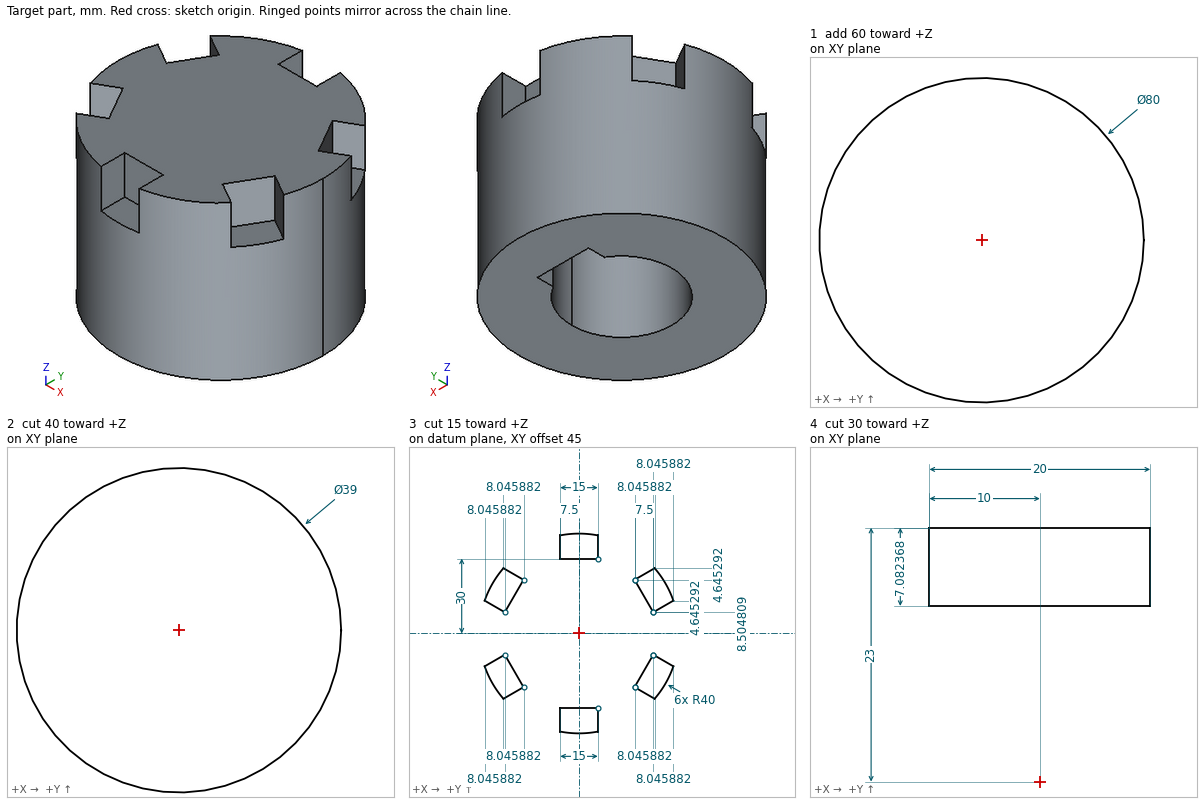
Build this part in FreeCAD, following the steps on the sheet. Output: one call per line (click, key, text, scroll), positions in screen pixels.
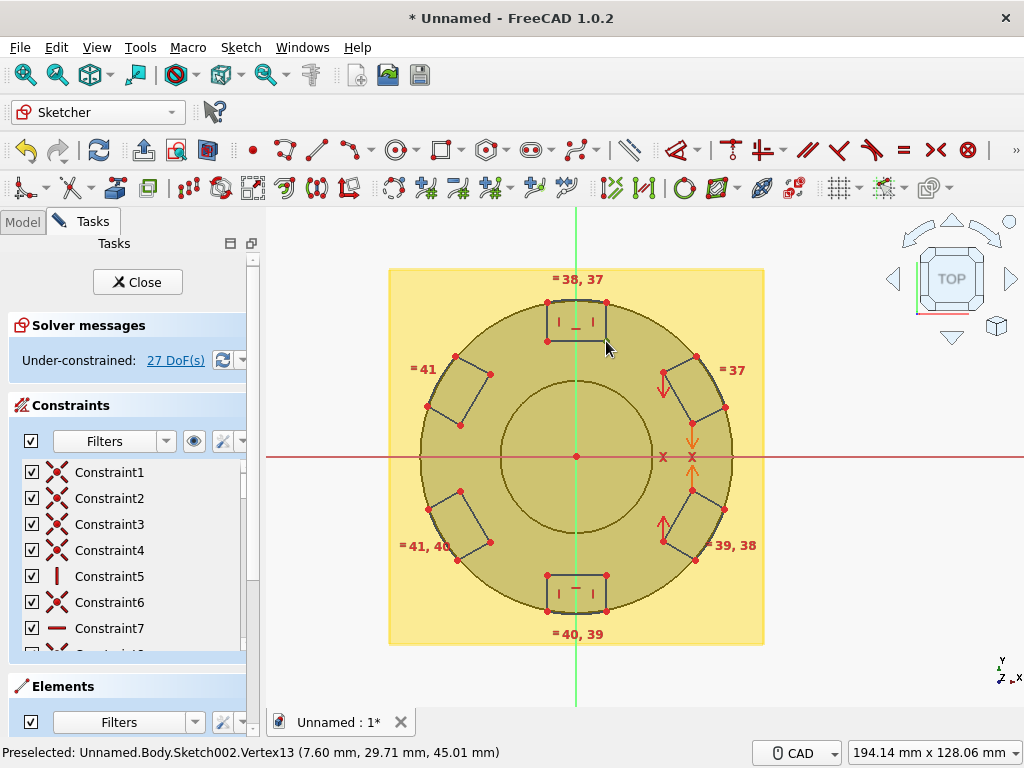
click(606, 575)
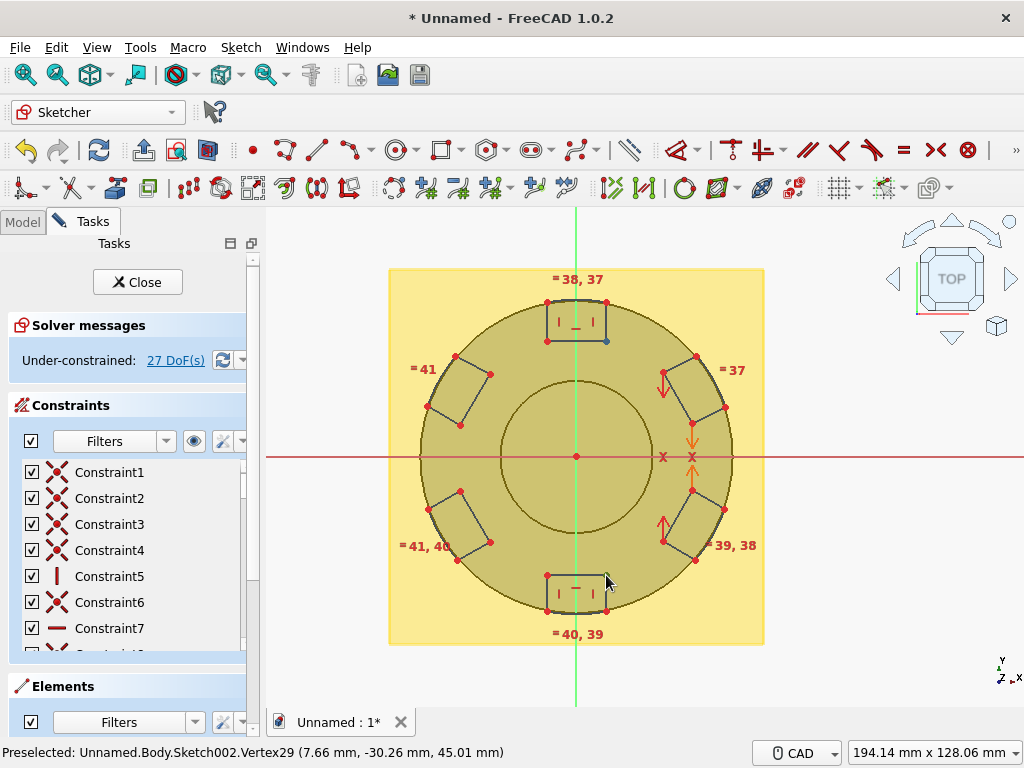
click(334, 457)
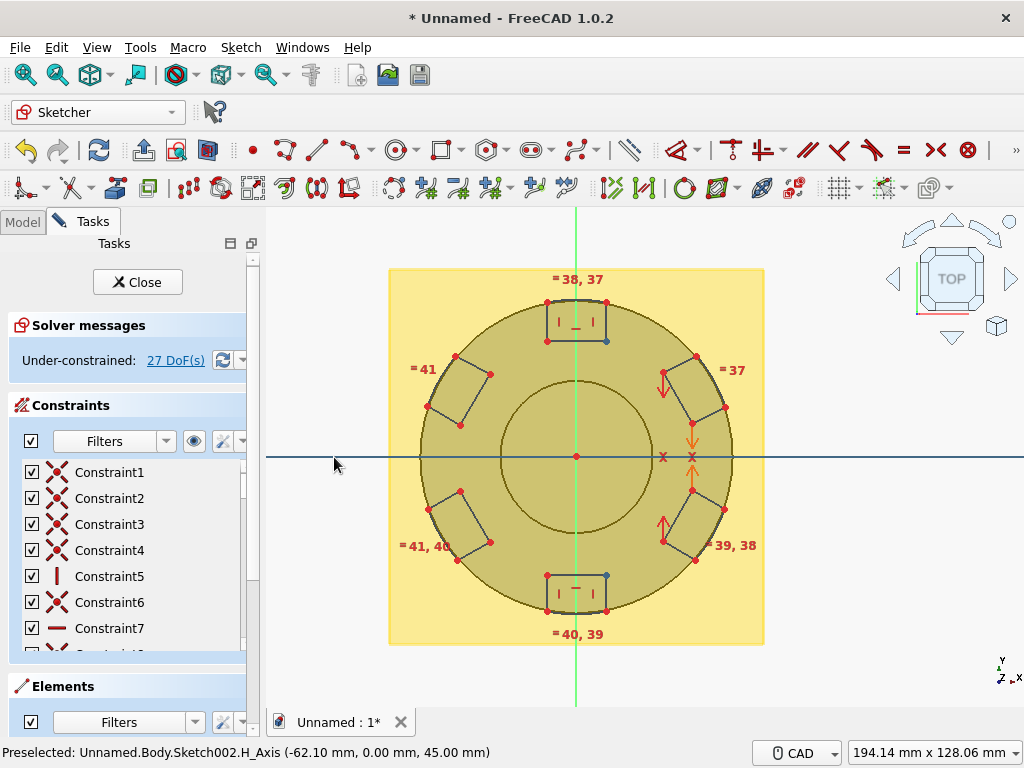
click(936, 150)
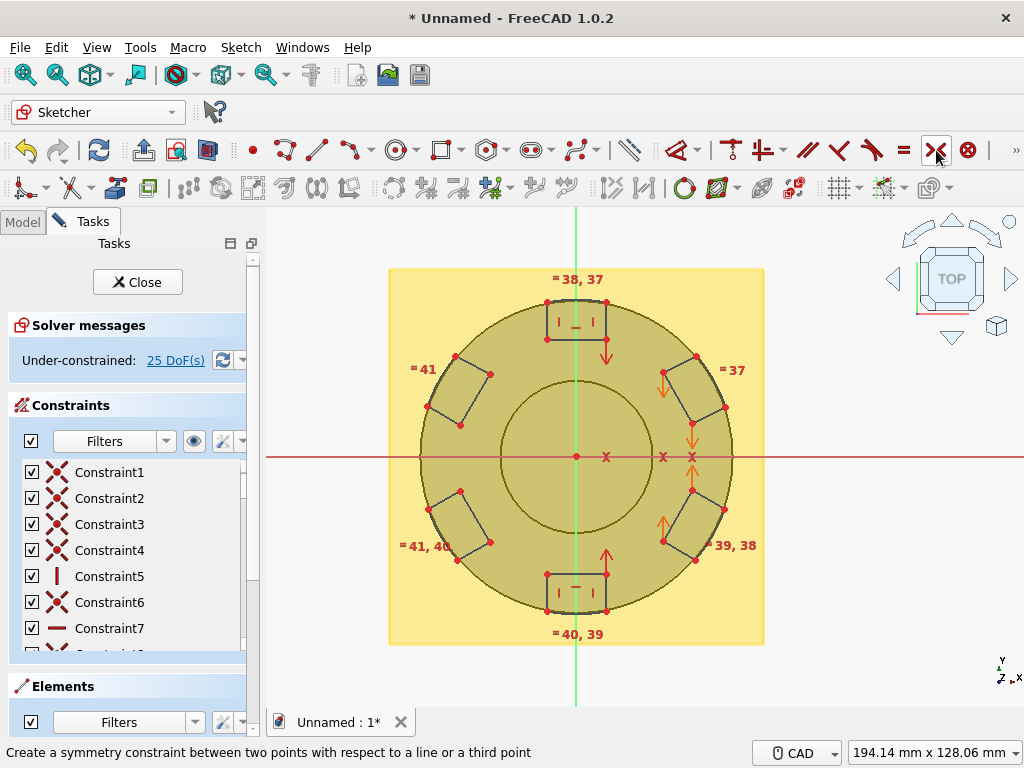
click(663, 541)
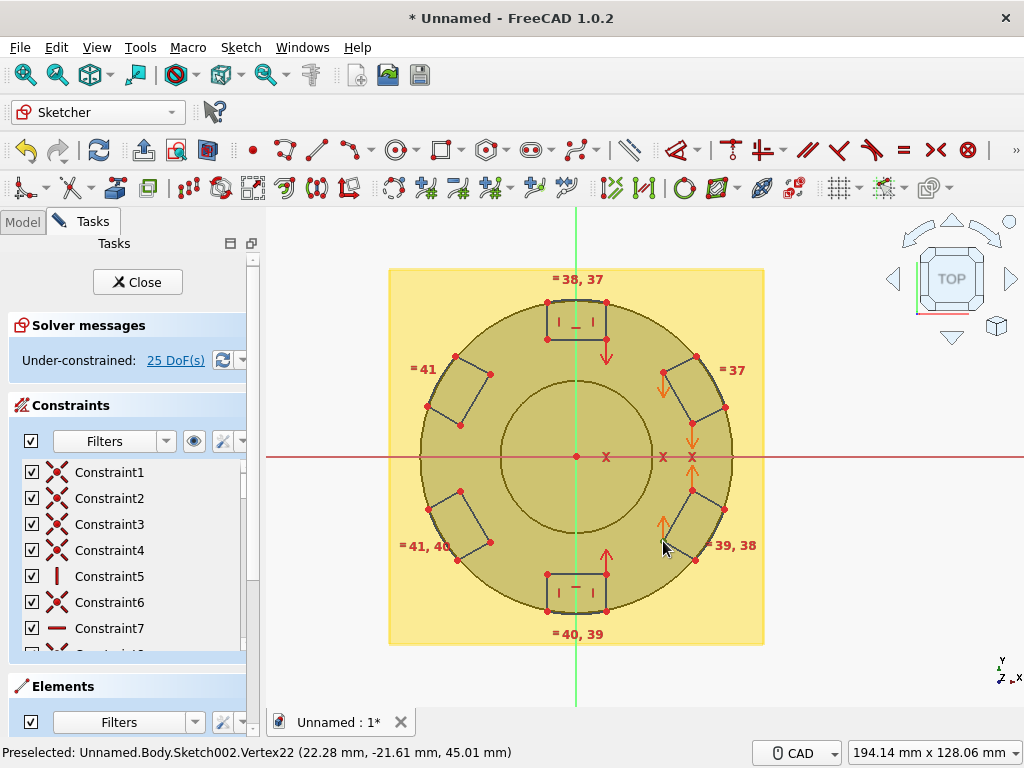
click(490, 542)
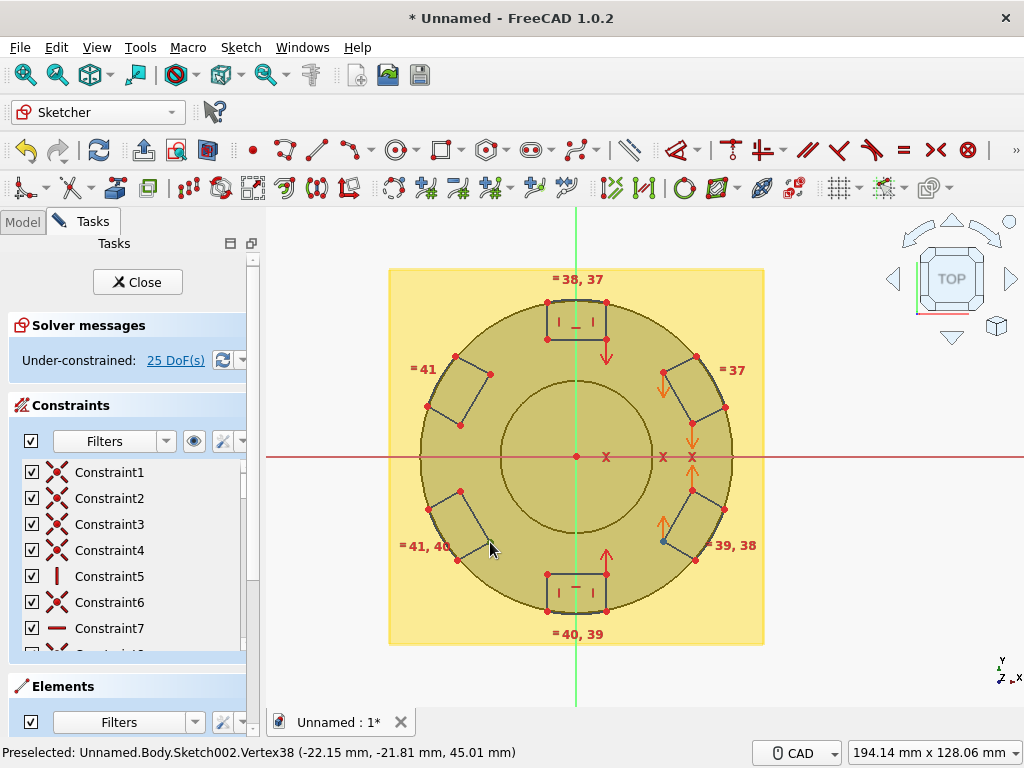
click(576, 647)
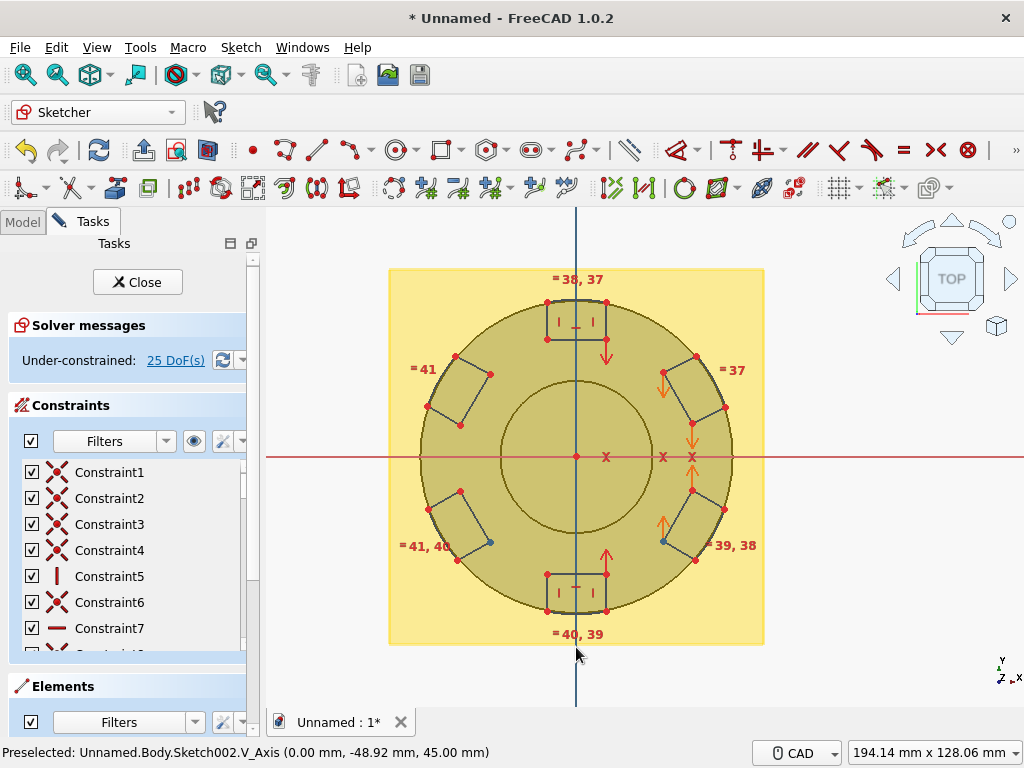
key(s)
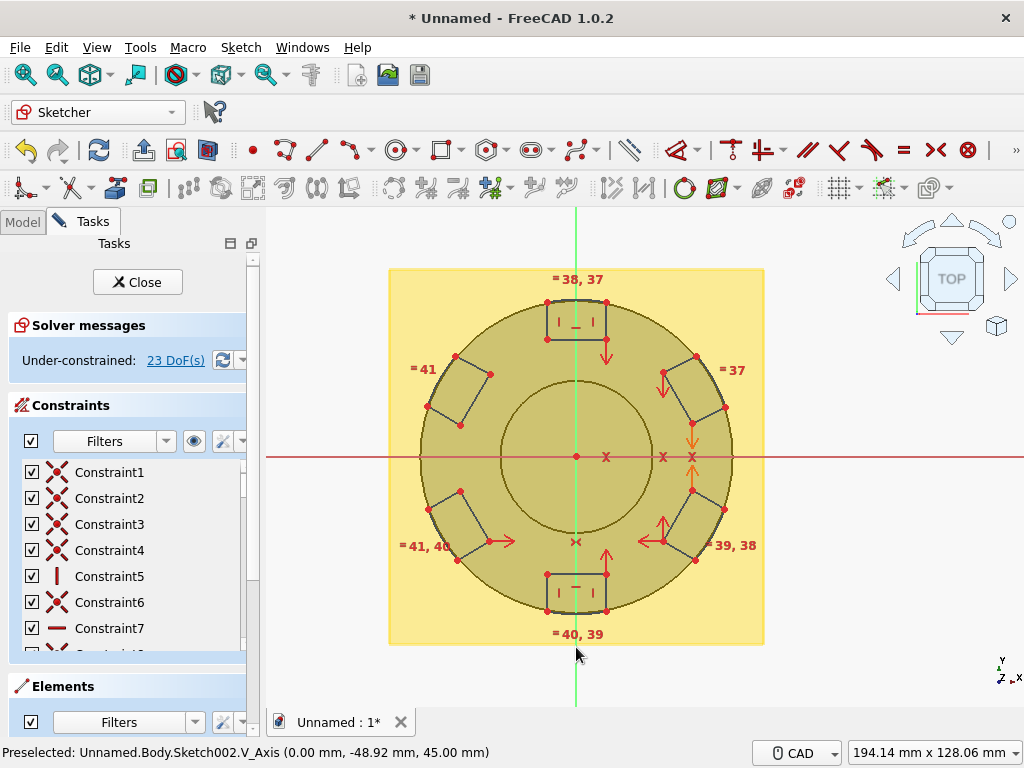
click(692, 490)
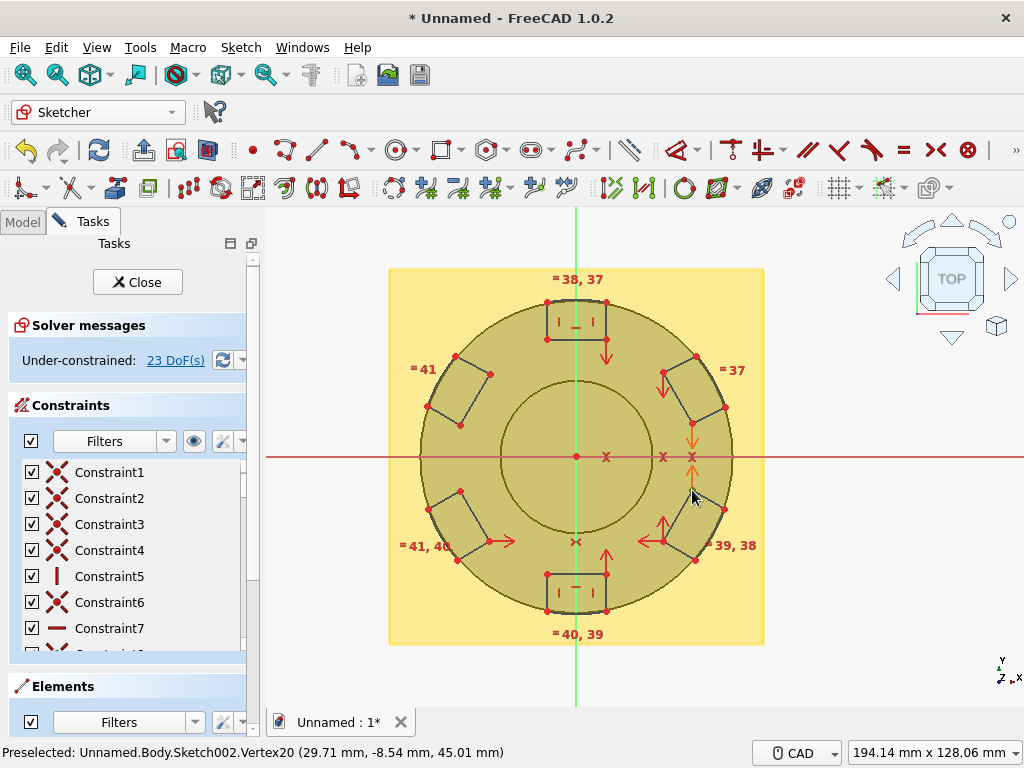
click(460, 491)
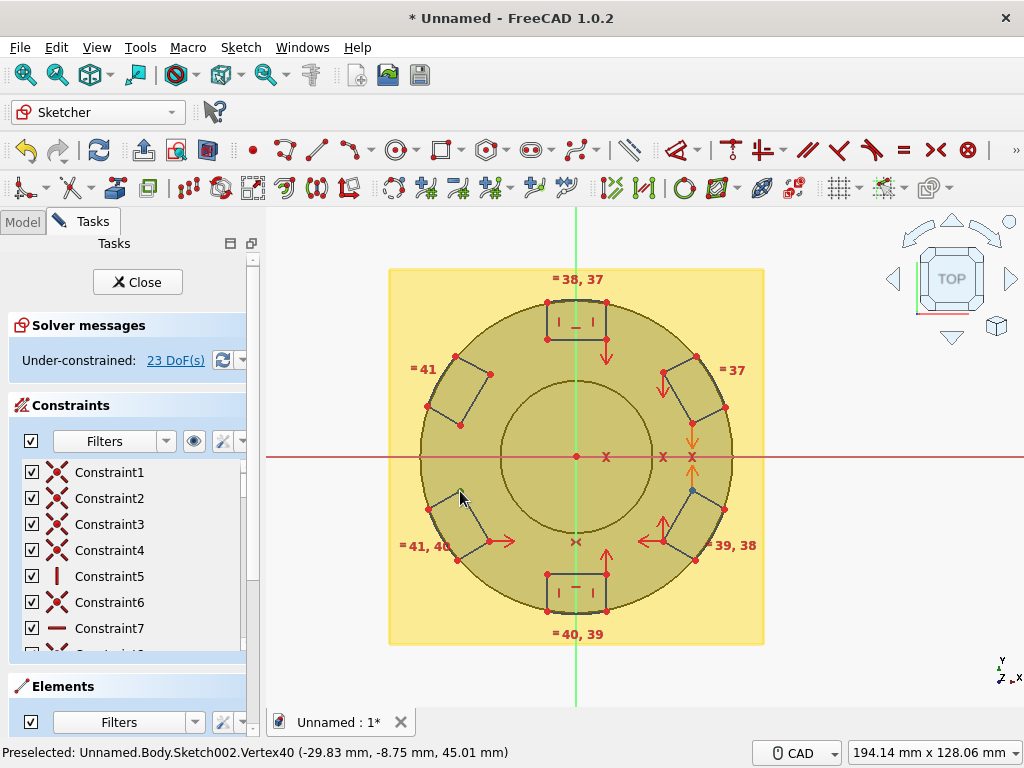
click(576, 647)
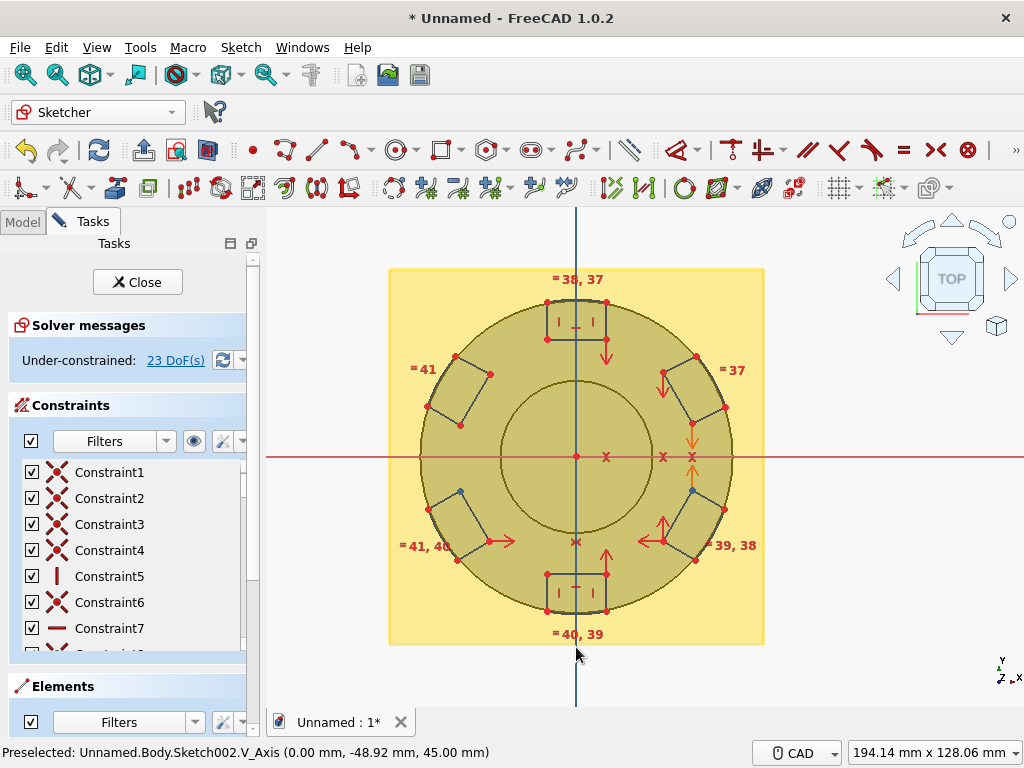
key(s)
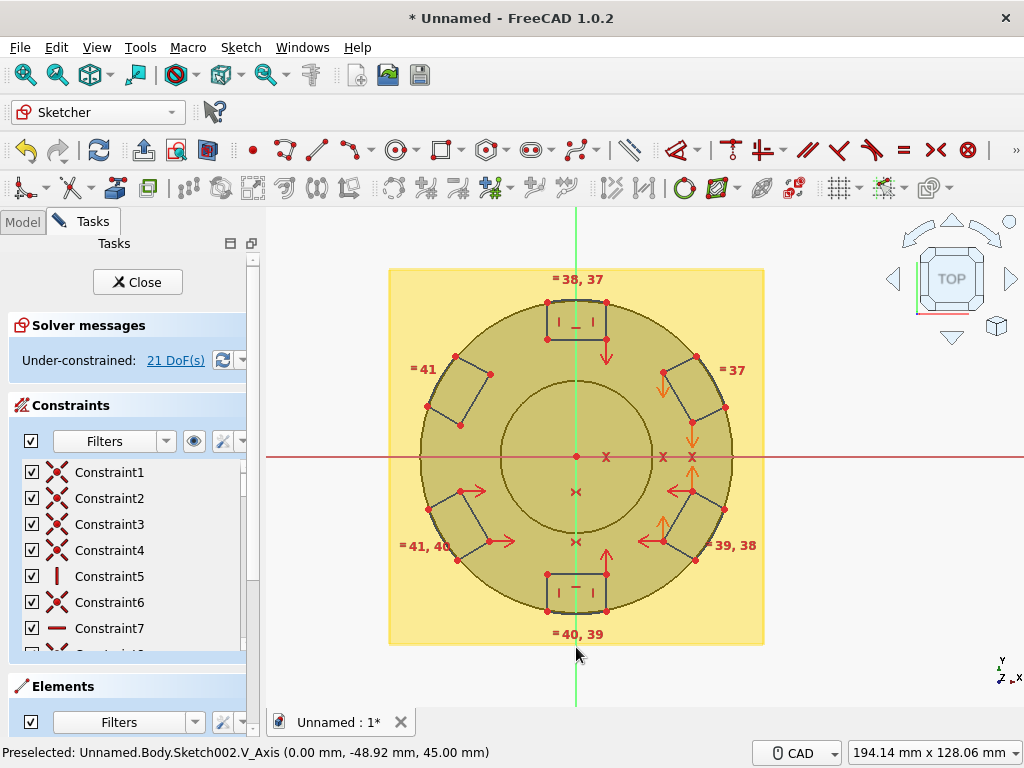
click(692, 423)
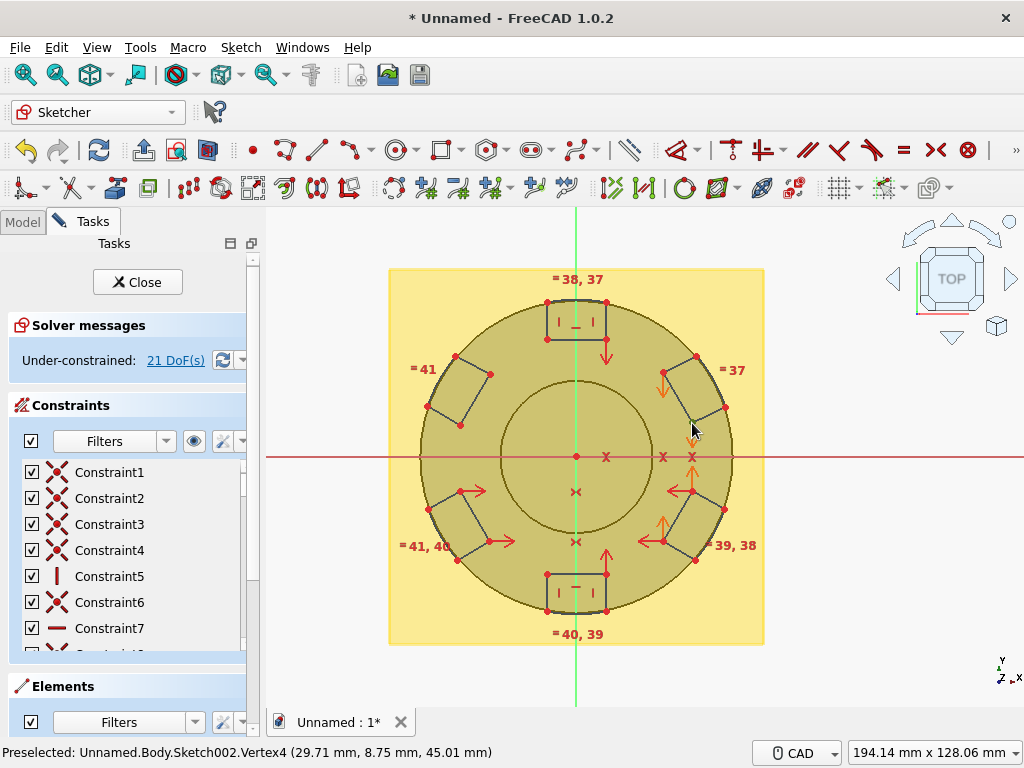
click(460, 425)